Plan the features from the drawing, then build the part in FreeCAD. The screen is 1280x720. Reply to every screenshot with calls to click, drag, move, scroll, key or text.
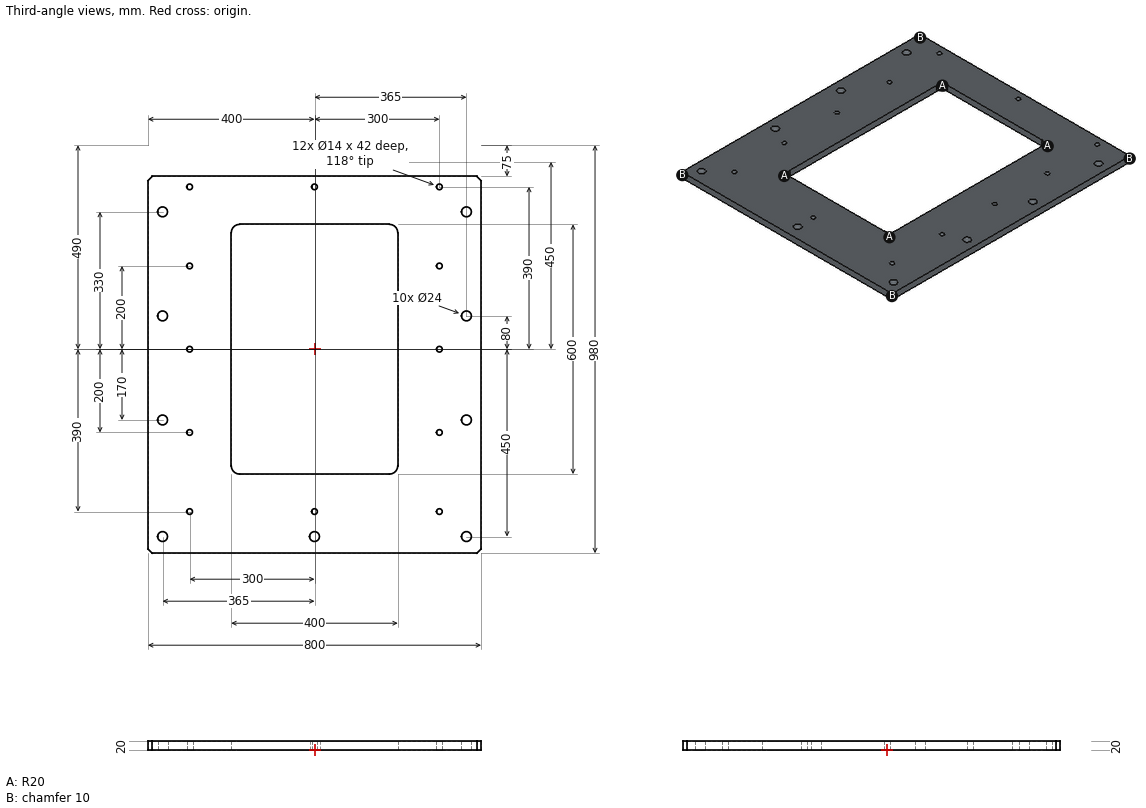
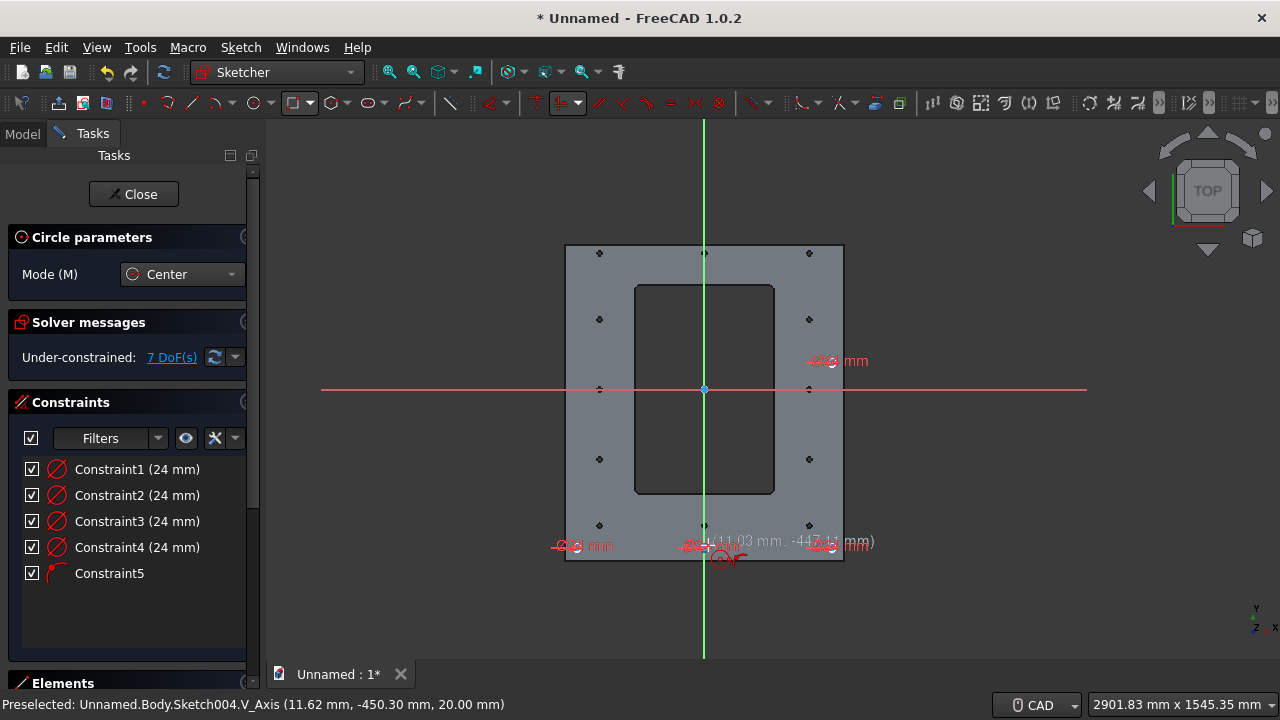
scroll(704, 232, up, 9)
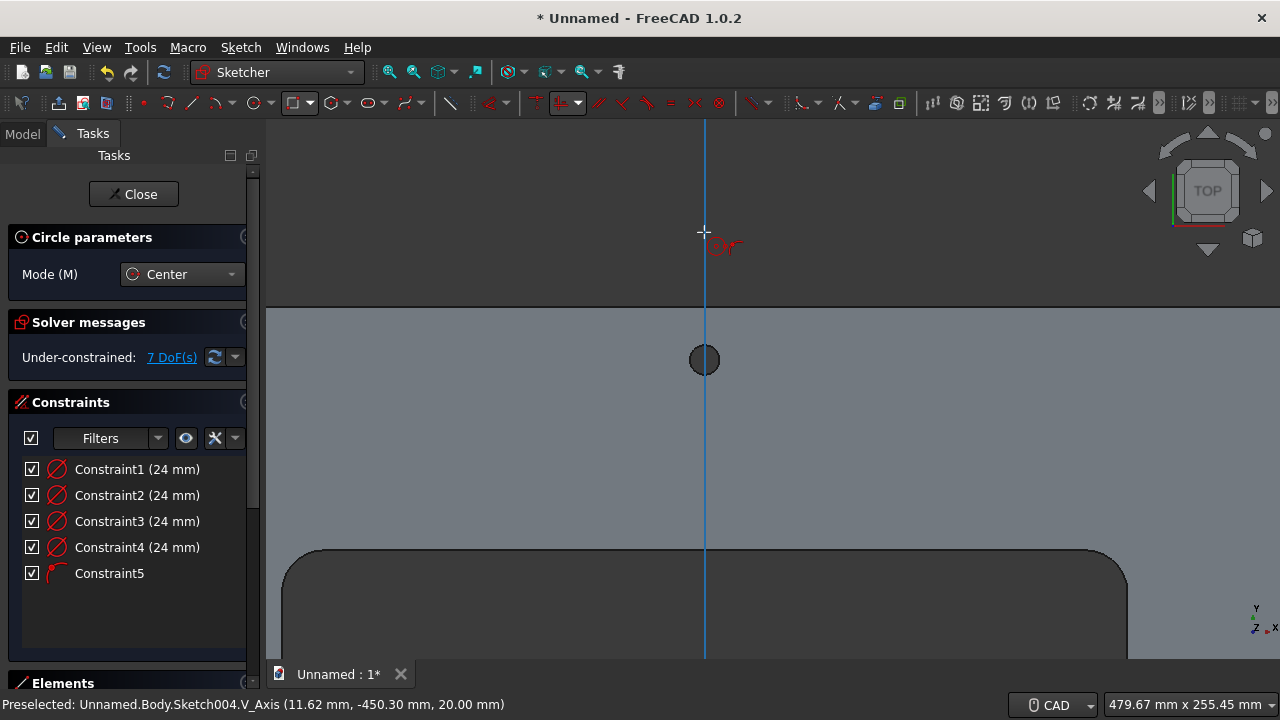
scroll(704, 231, down, 9)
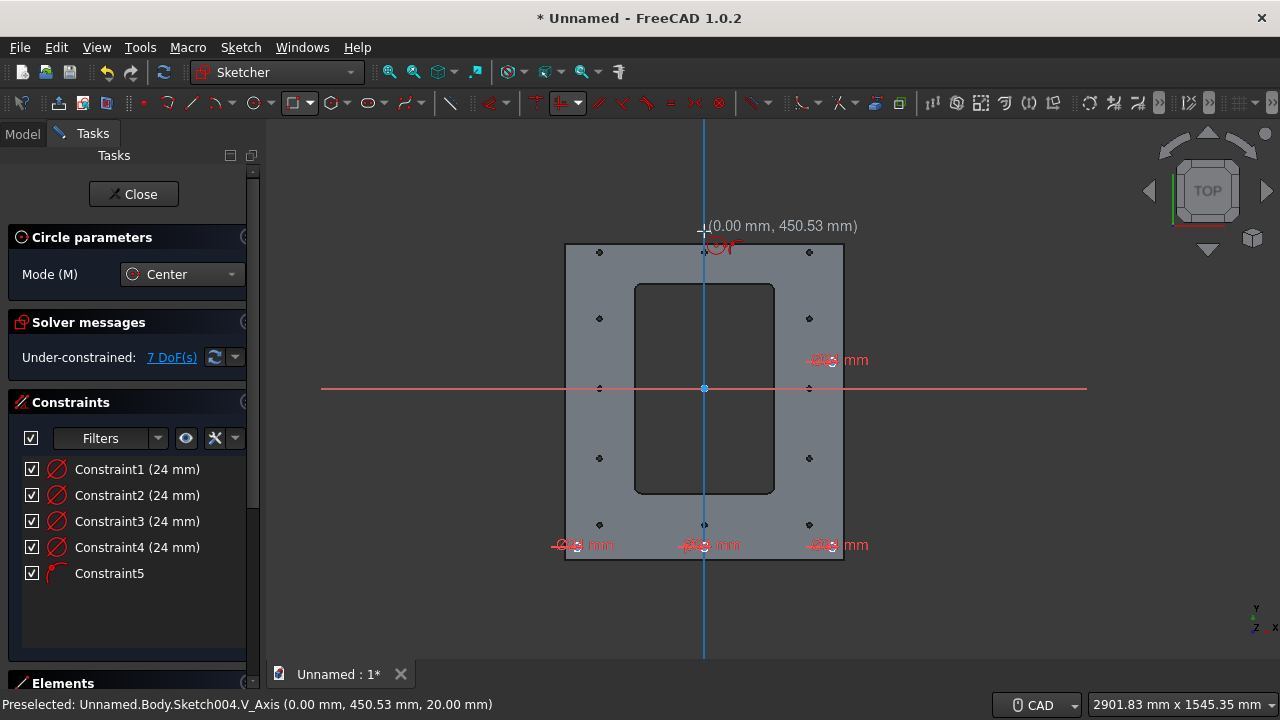
click(704, 232)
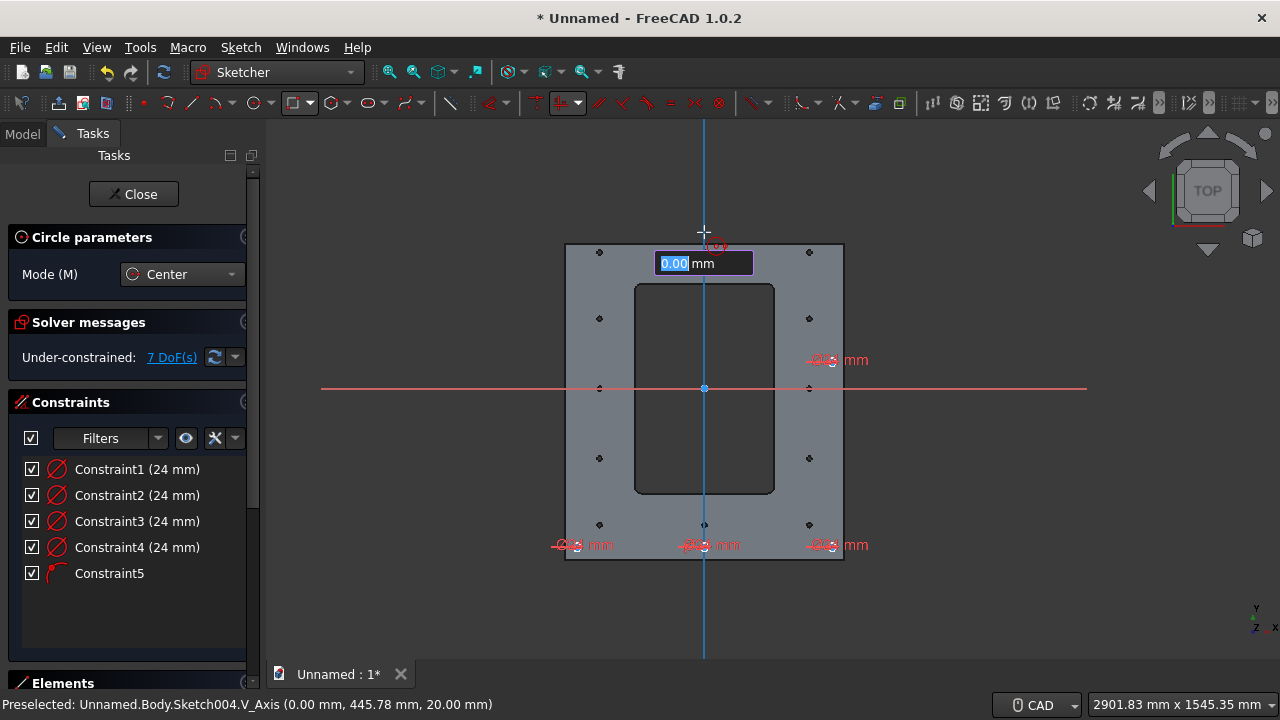
scroll(708, 230, up, 7)
move(708, 230)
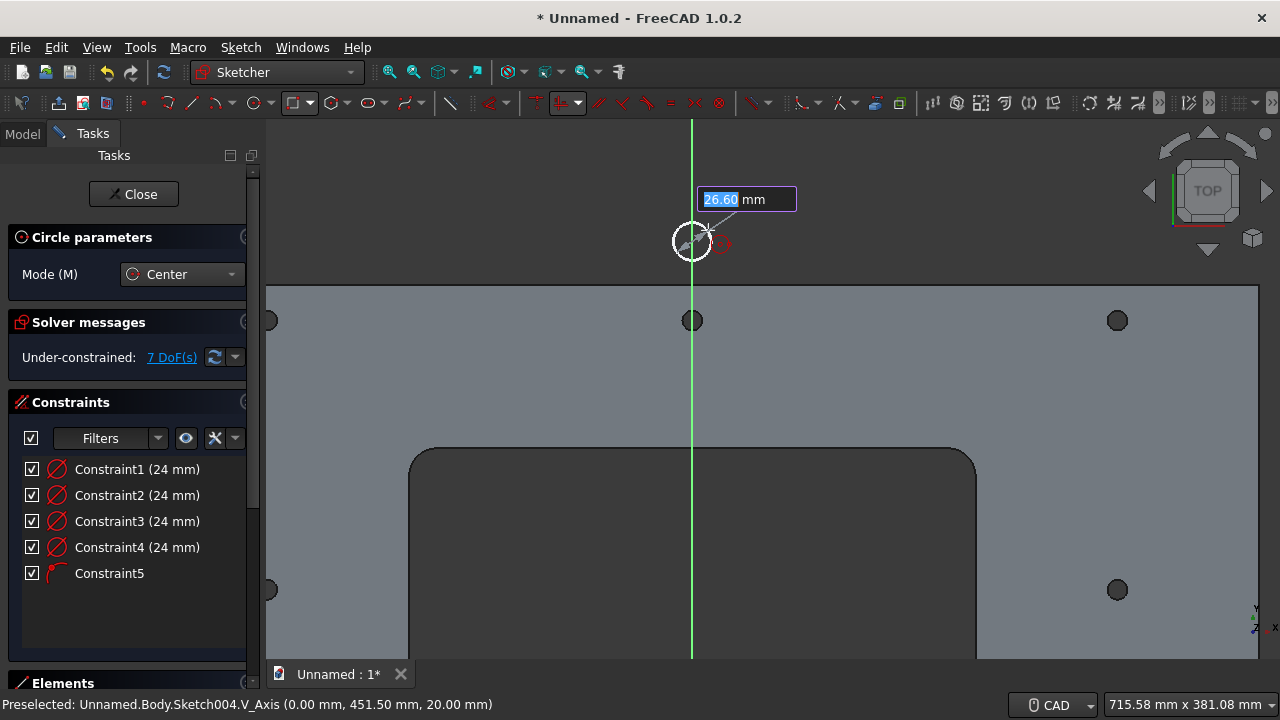
text(24)
key(Return)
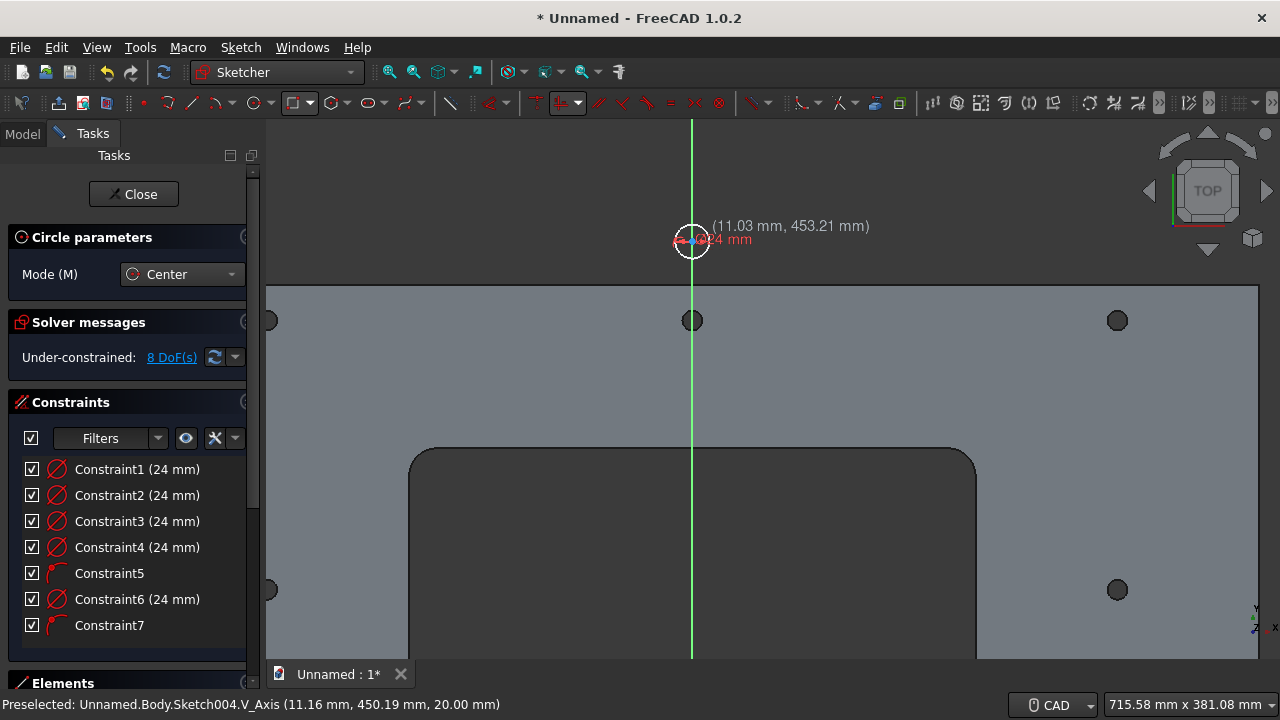
scroll(708, 231, down, 7)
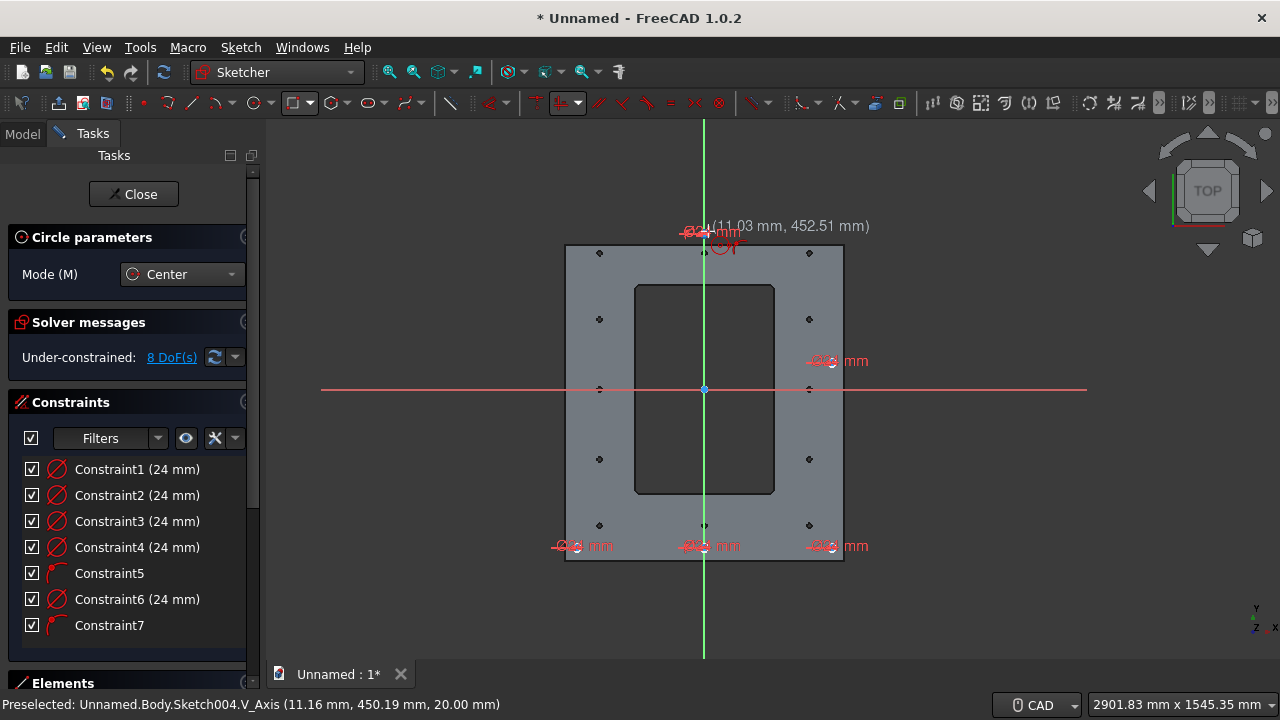
scroll(577, 274, up, 9)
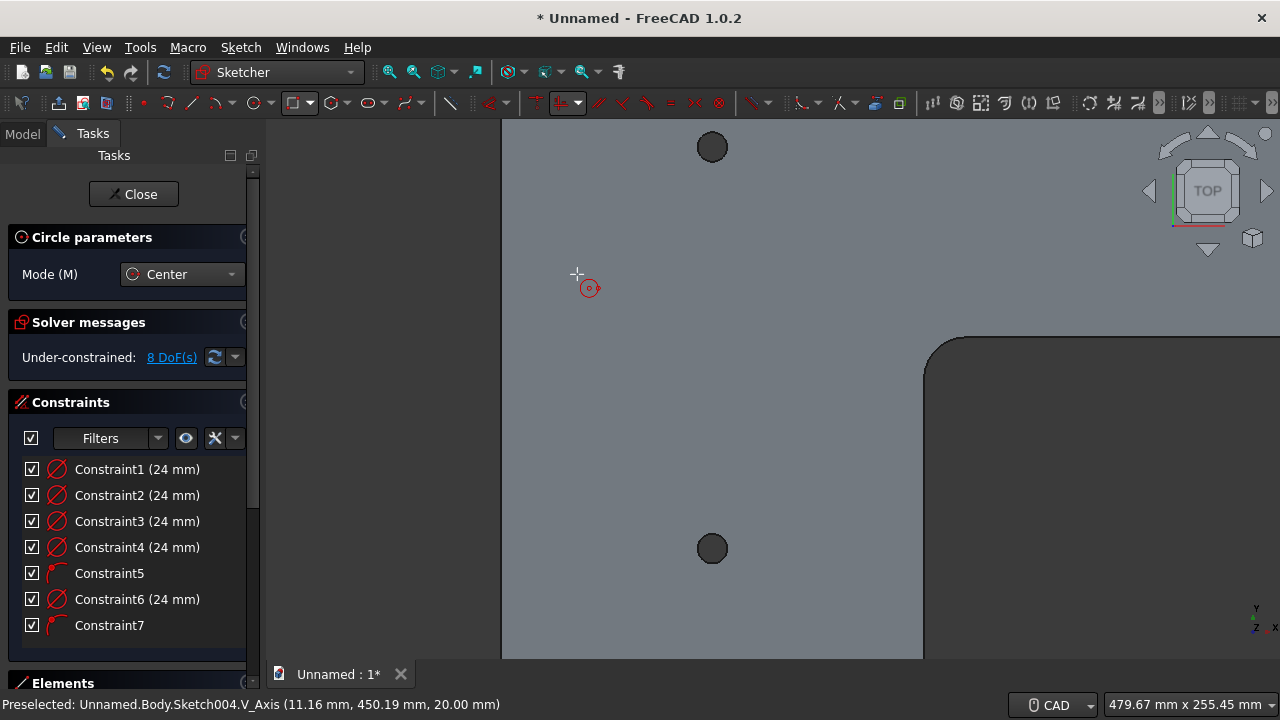
scroll(577, 274, down, 9)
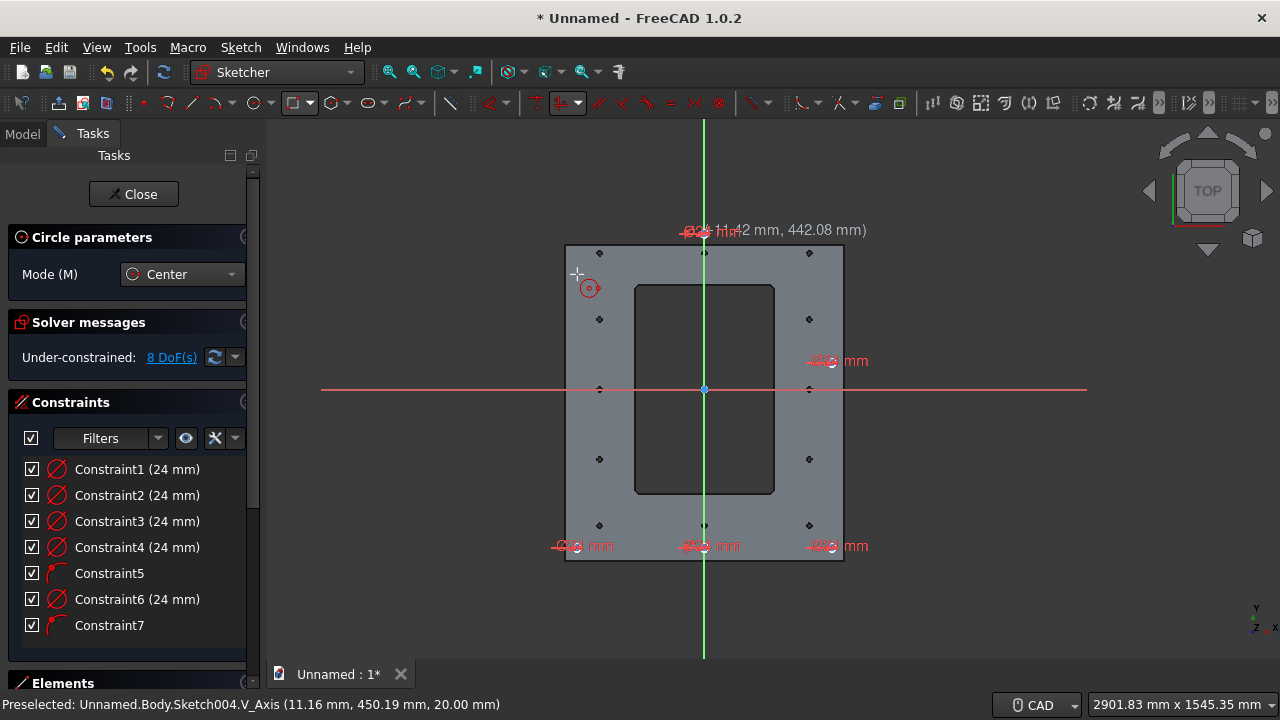
click(577, 274)
move(580, 271)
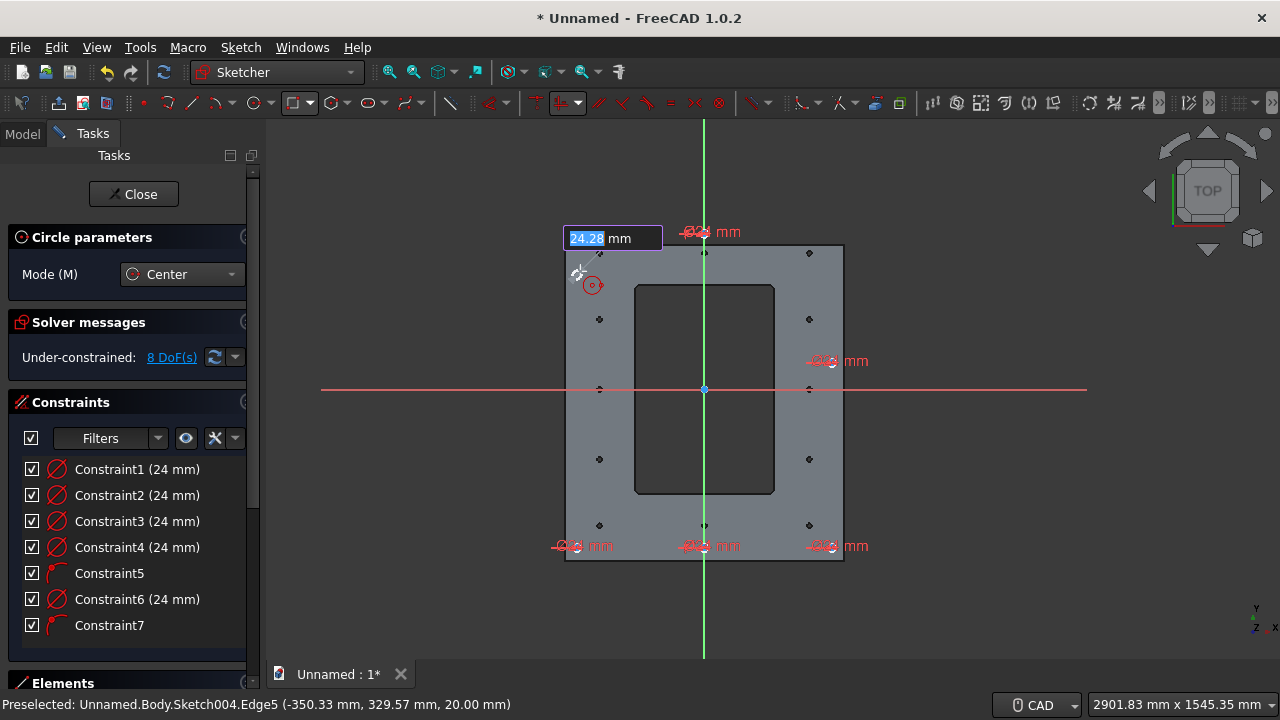
text(24)
key(Return)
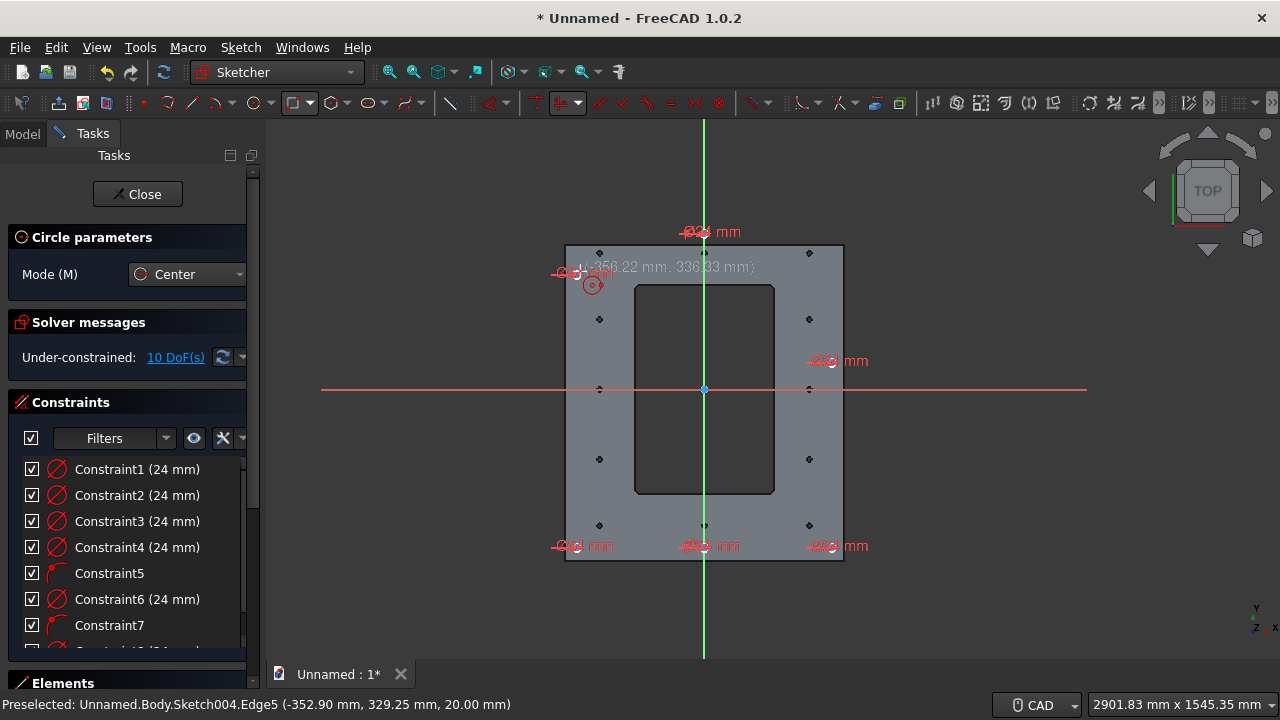
scroll(832, 274, up, 9)